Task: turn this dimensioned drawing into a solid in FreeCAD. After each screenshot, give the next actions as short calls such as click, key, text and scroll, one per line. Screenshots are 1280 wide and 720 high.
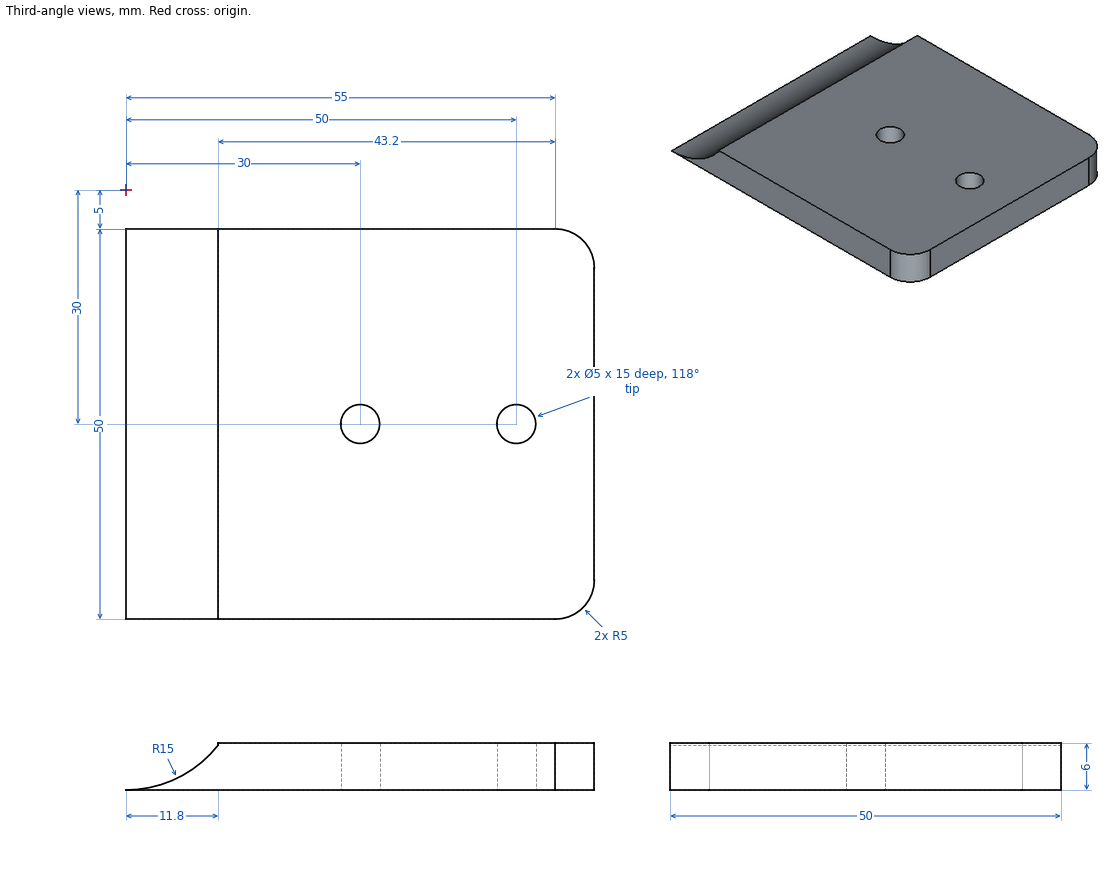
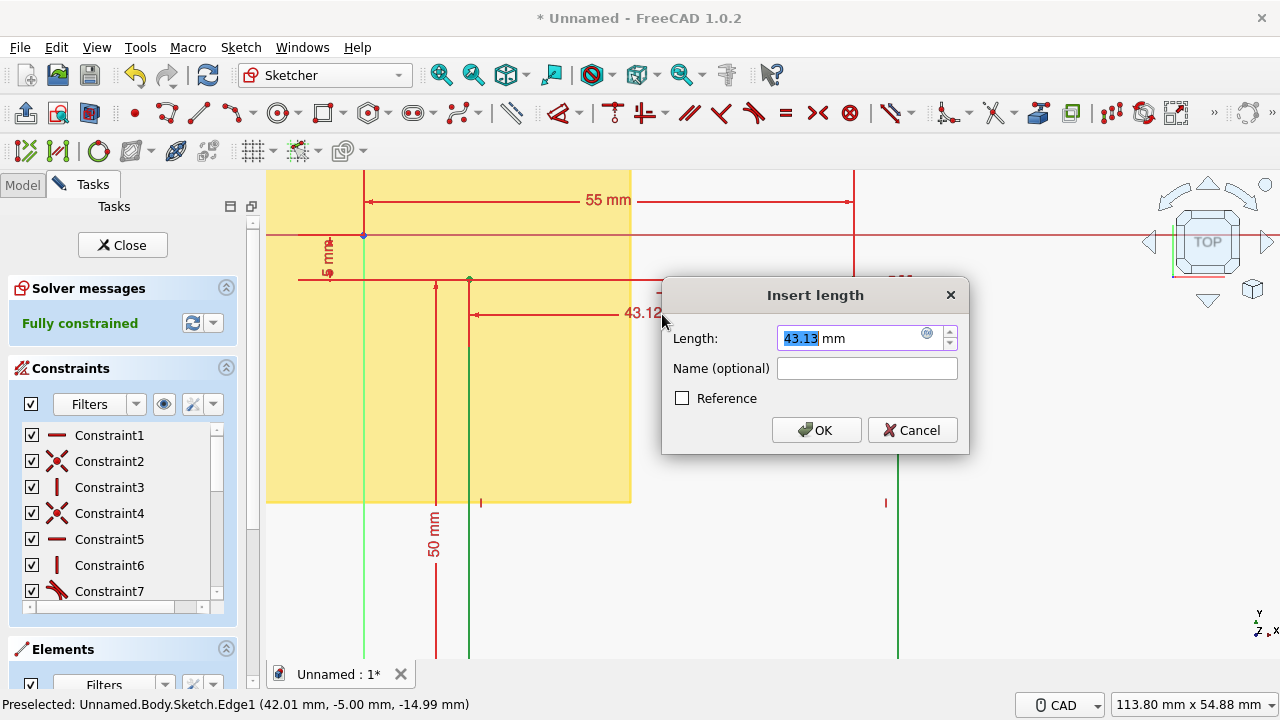
text(43.2)
key(Return)
key(Escape)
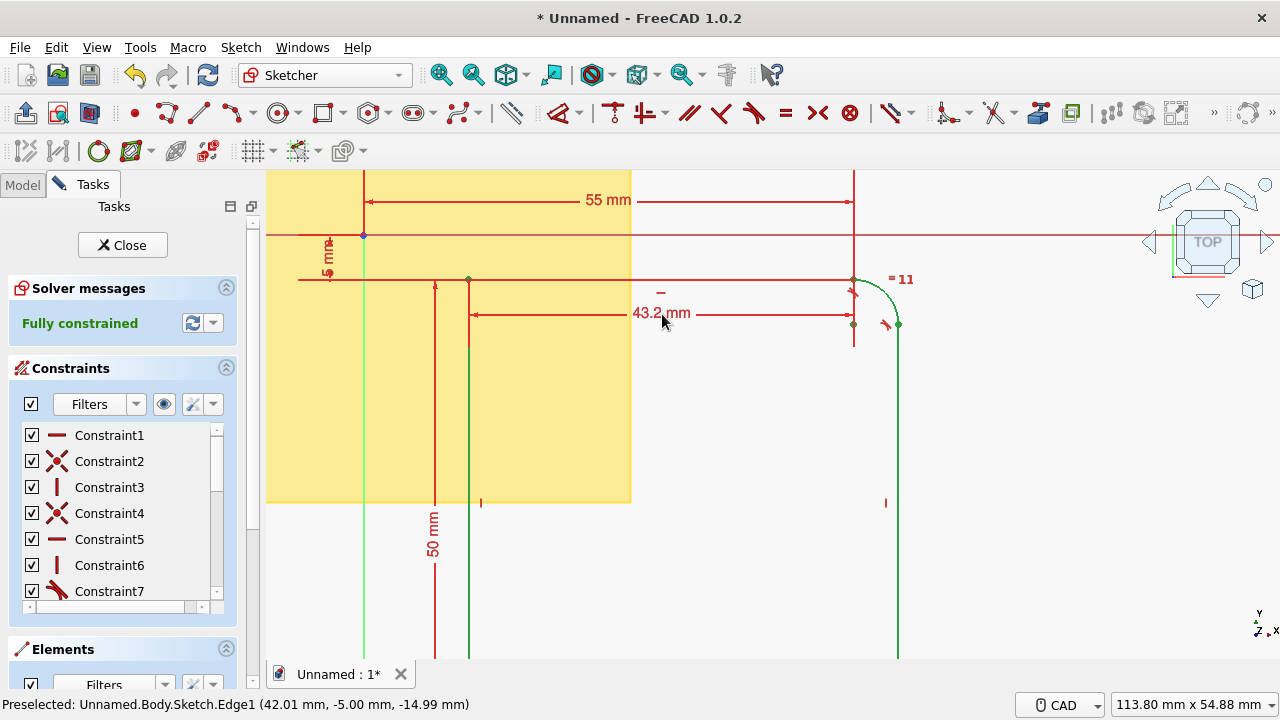
click(123, 245)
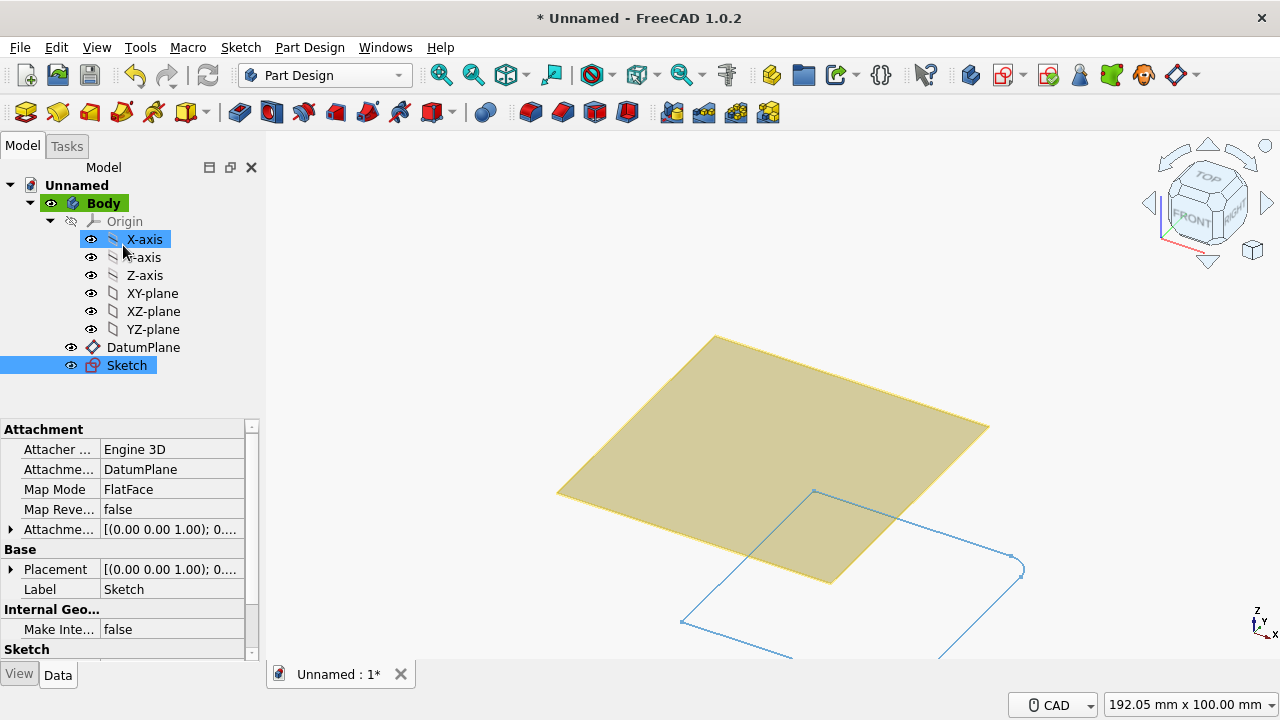
click(26, 112)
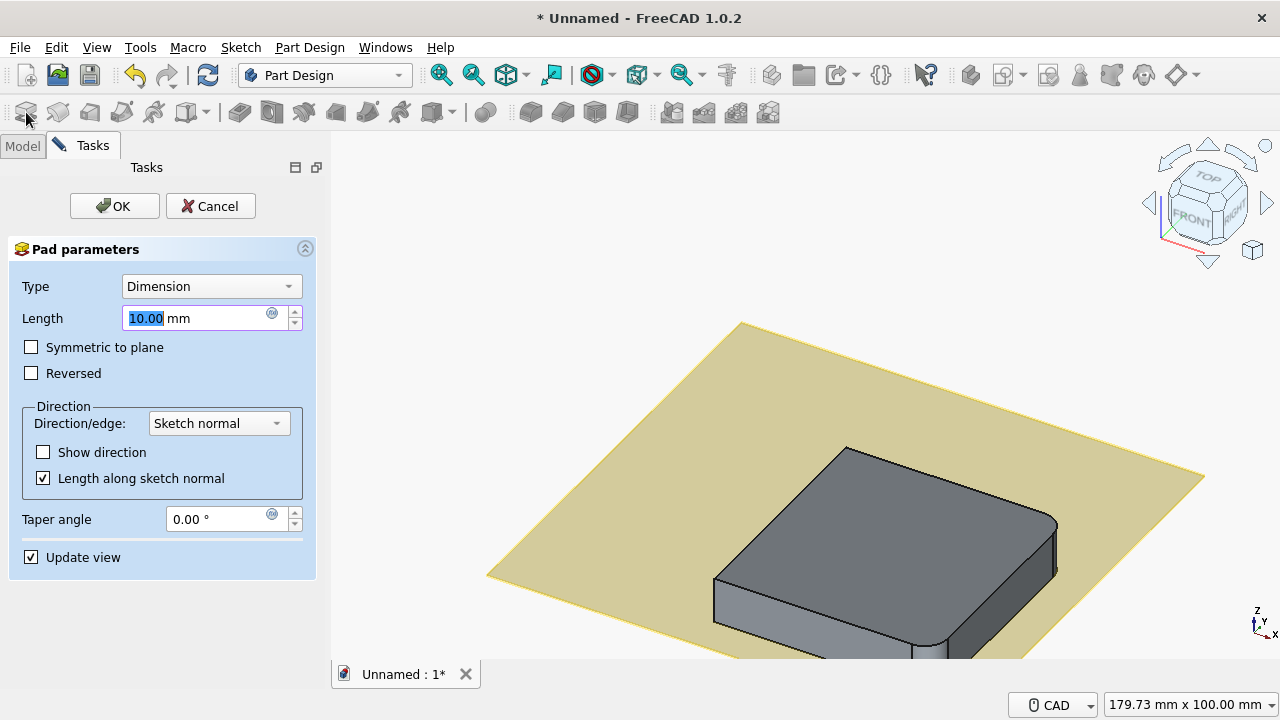
text(6)
key(Tab)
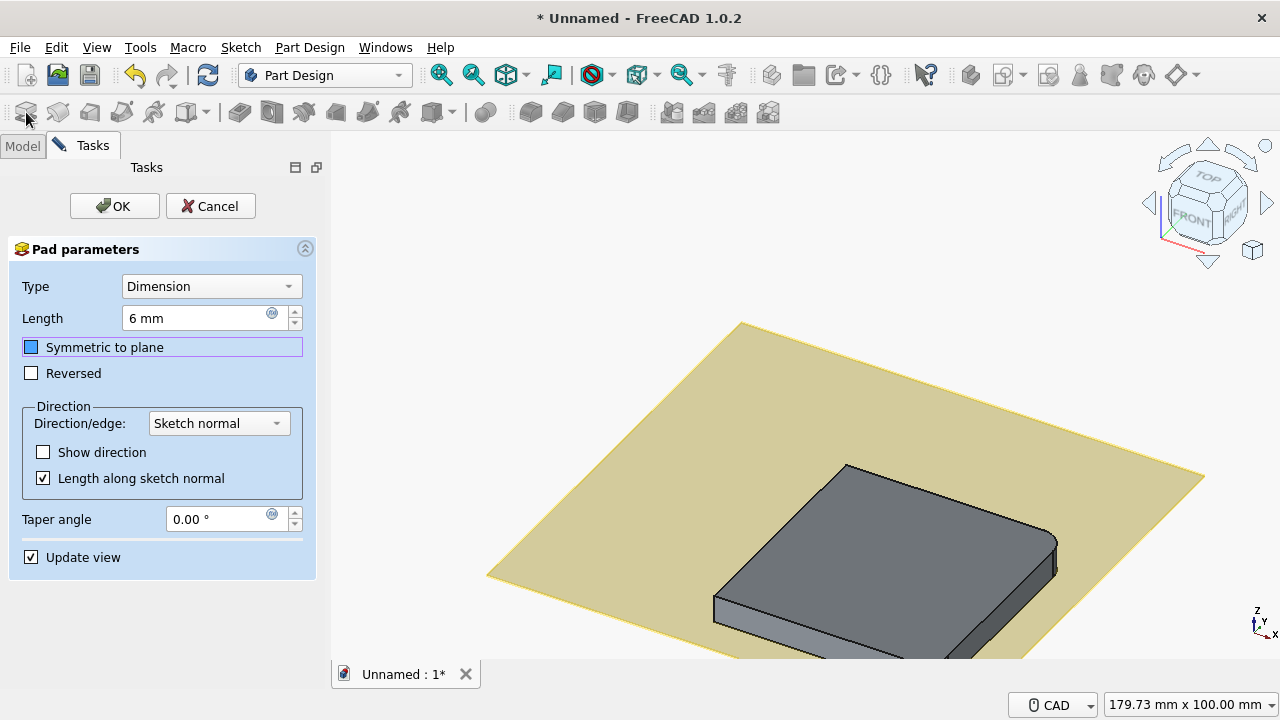
click(115, 206)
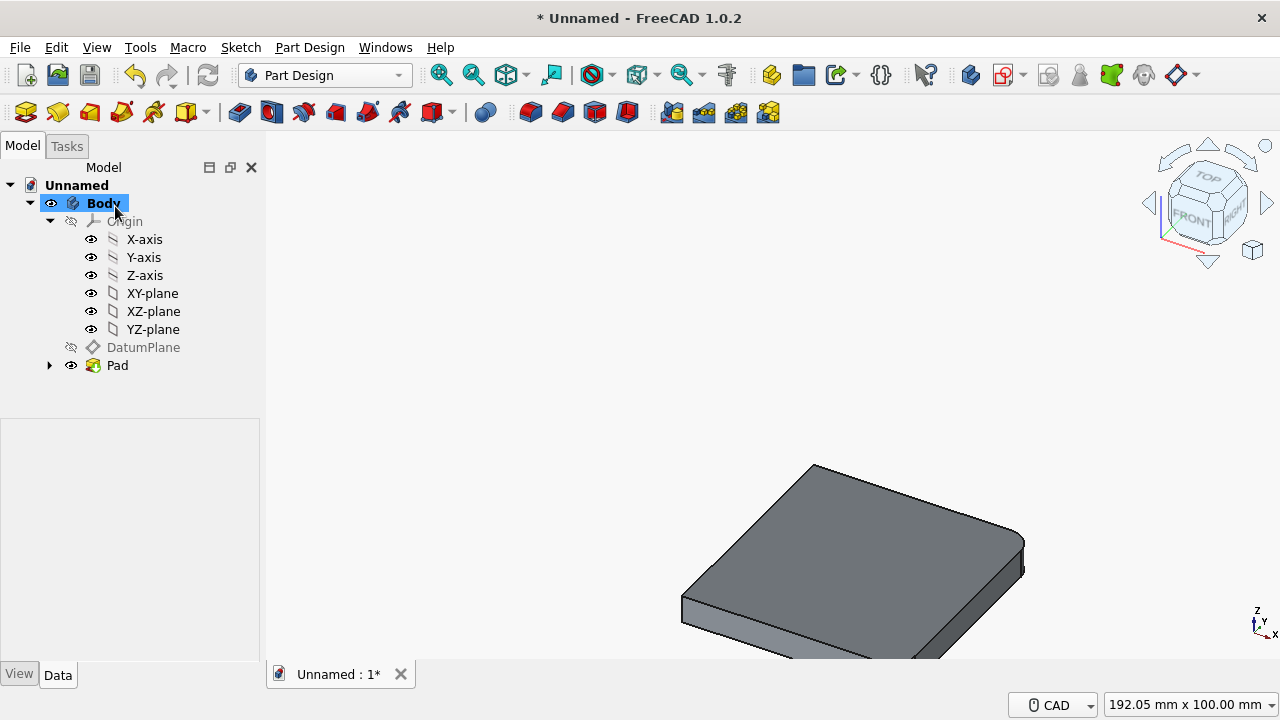
click(442, 76)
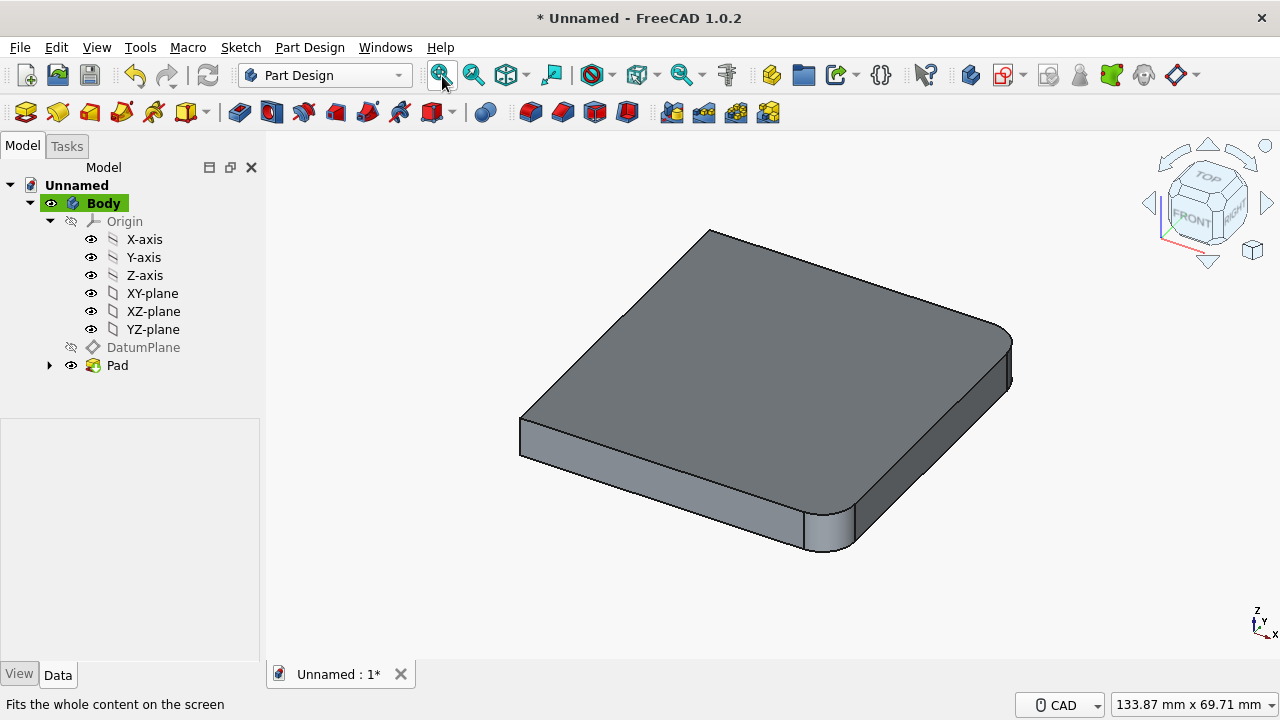
key(4)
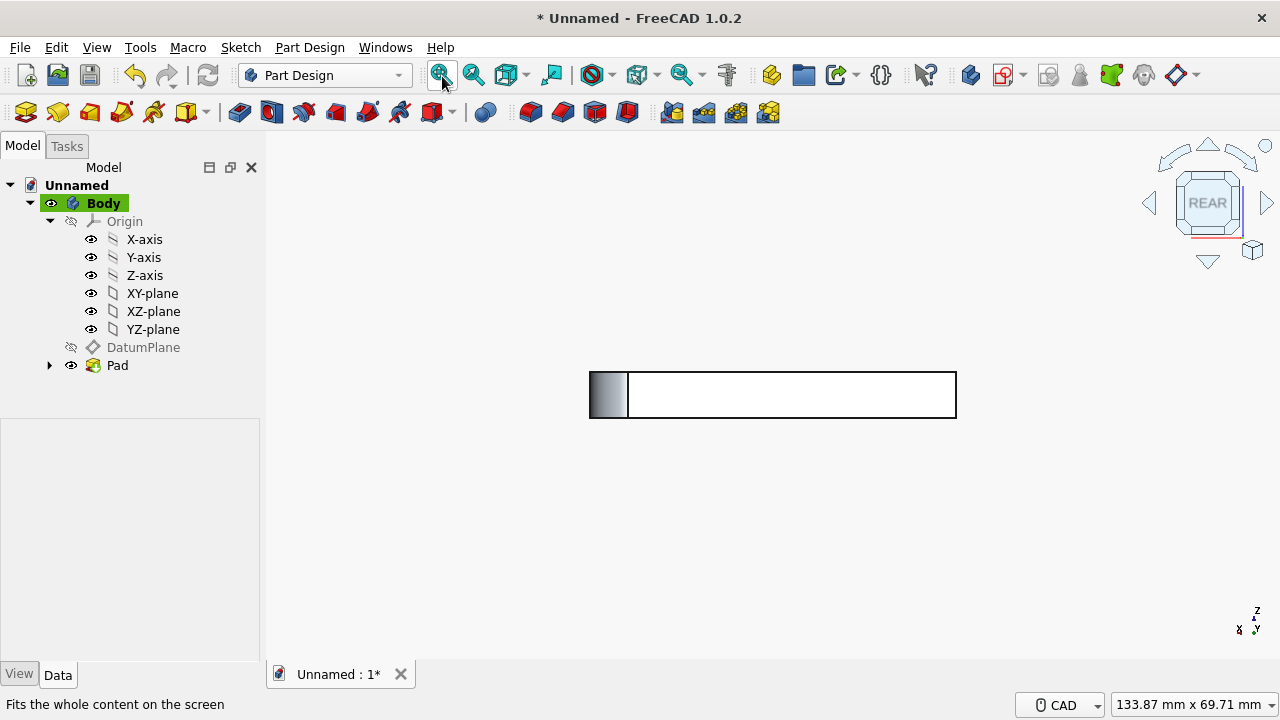
click(442, 76)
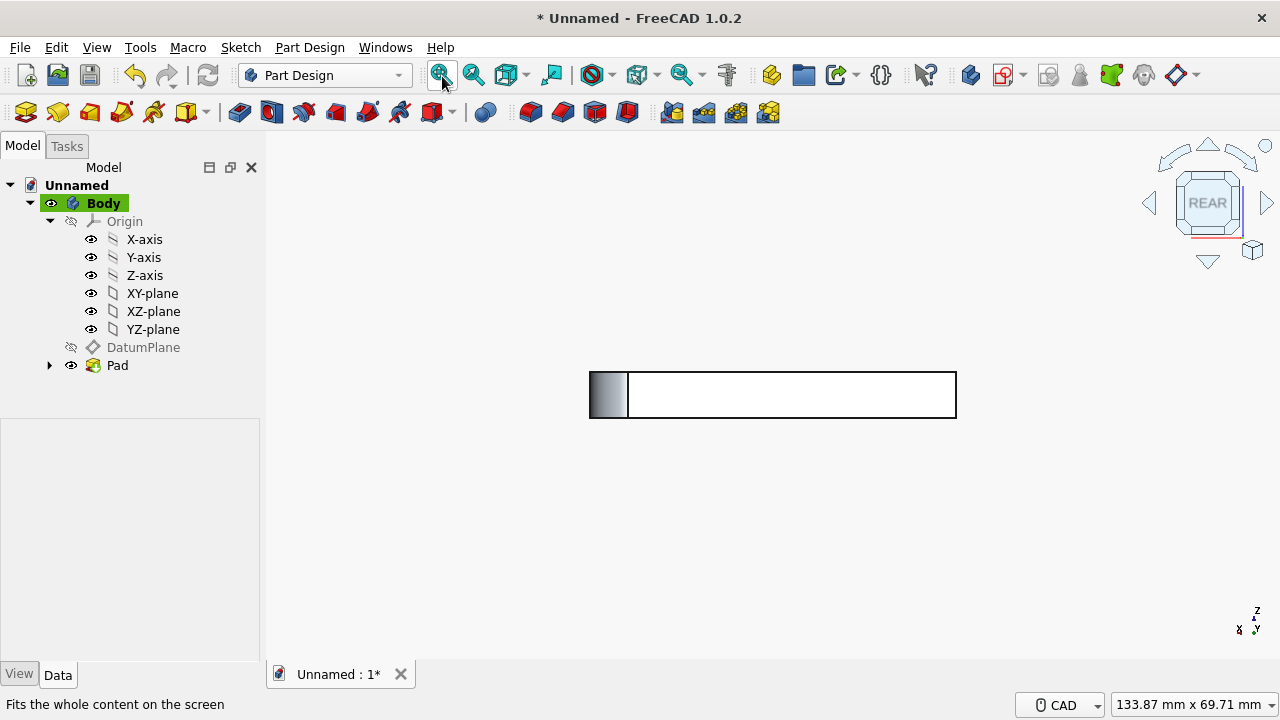
click(652, 394)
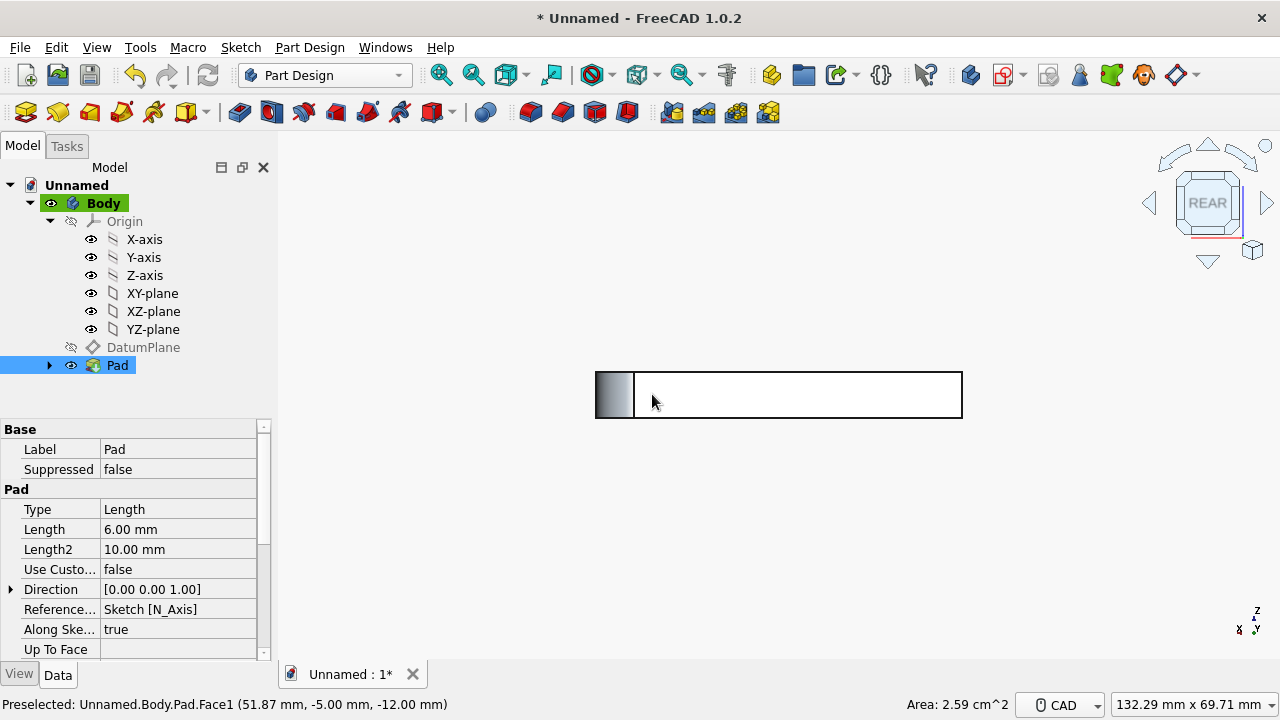
click(1004, 76)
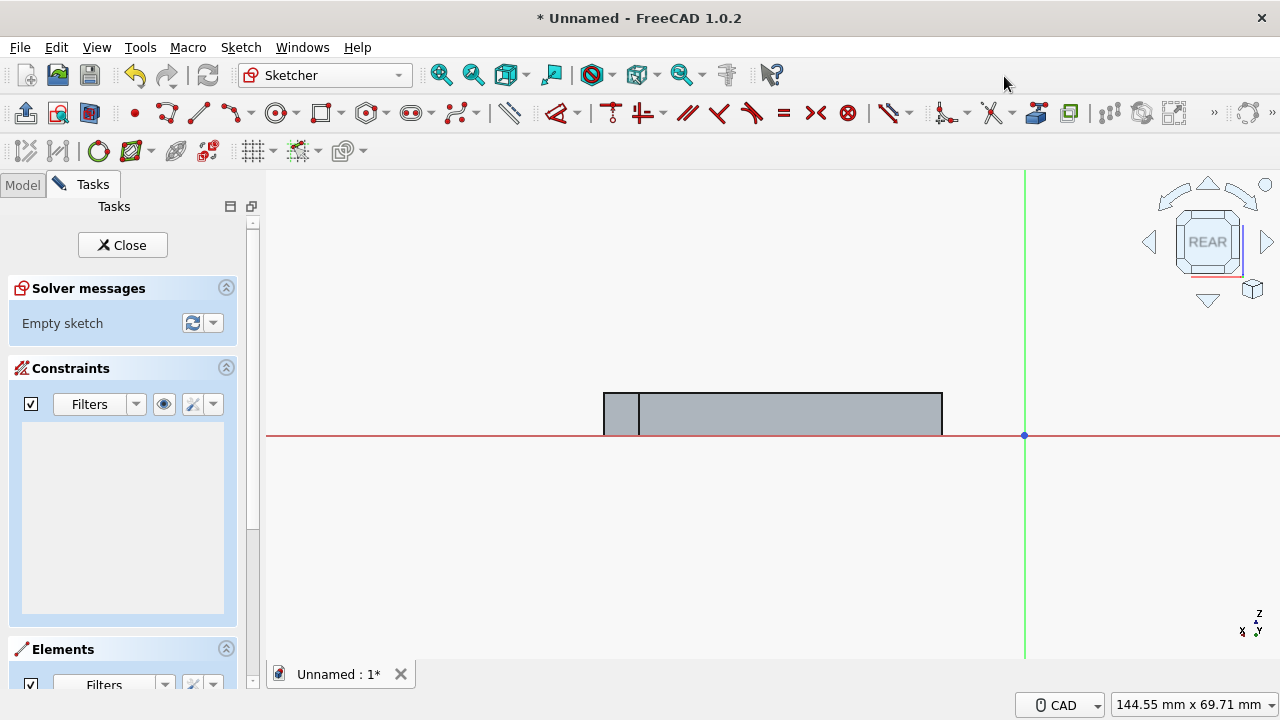
scroll(1027, 416, up, 10)